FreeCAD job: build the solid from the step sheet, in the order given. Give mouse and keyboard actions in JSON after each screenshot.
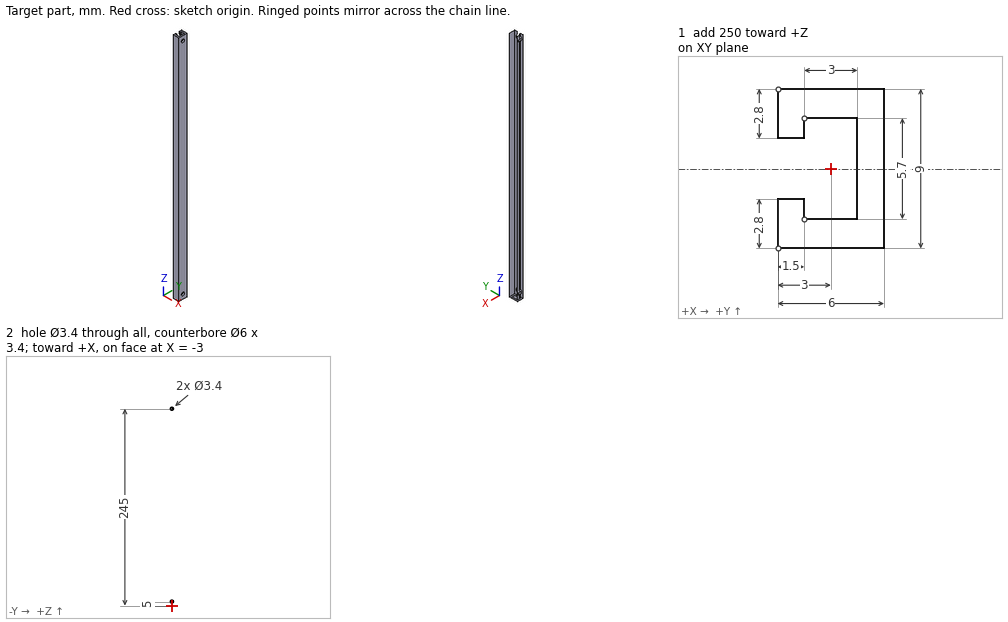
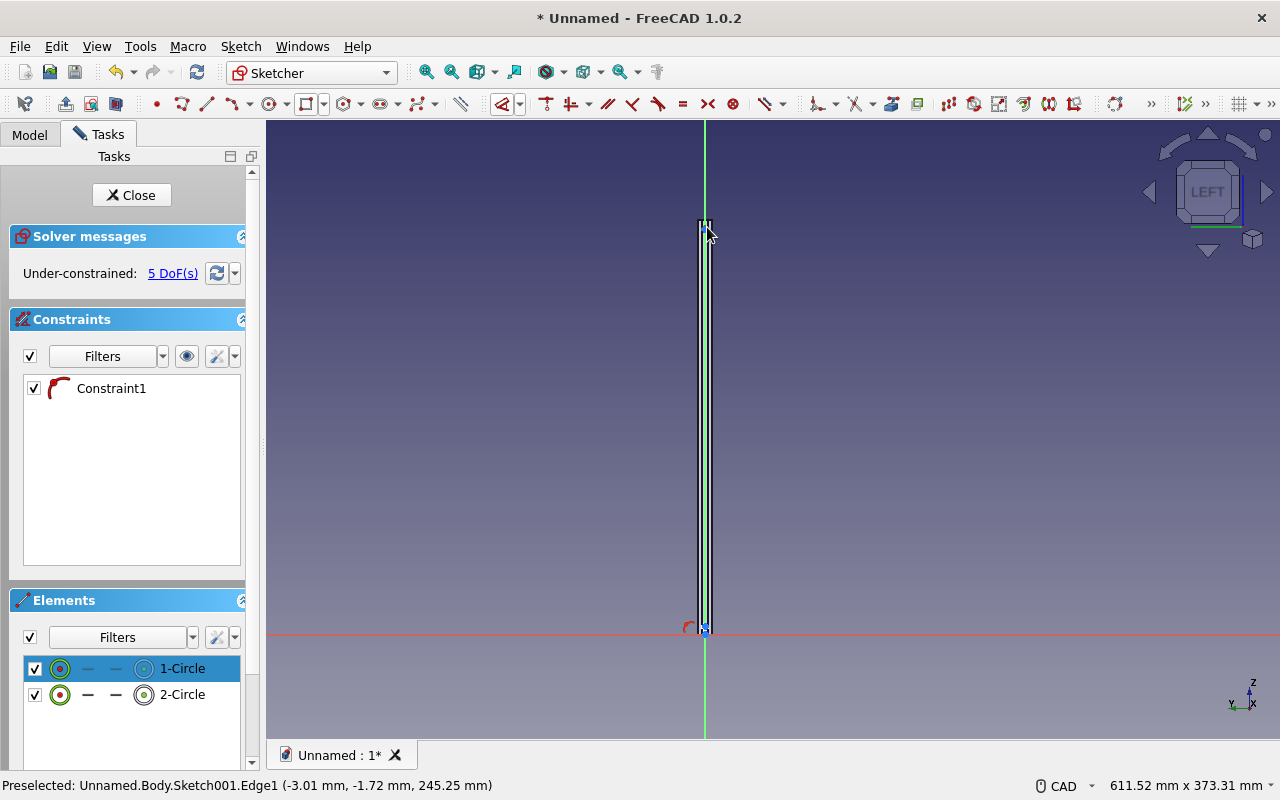
{"action": "scroll", "coordinate": [707, 625], "scroll_direction": "up", "scroll_amount": 10}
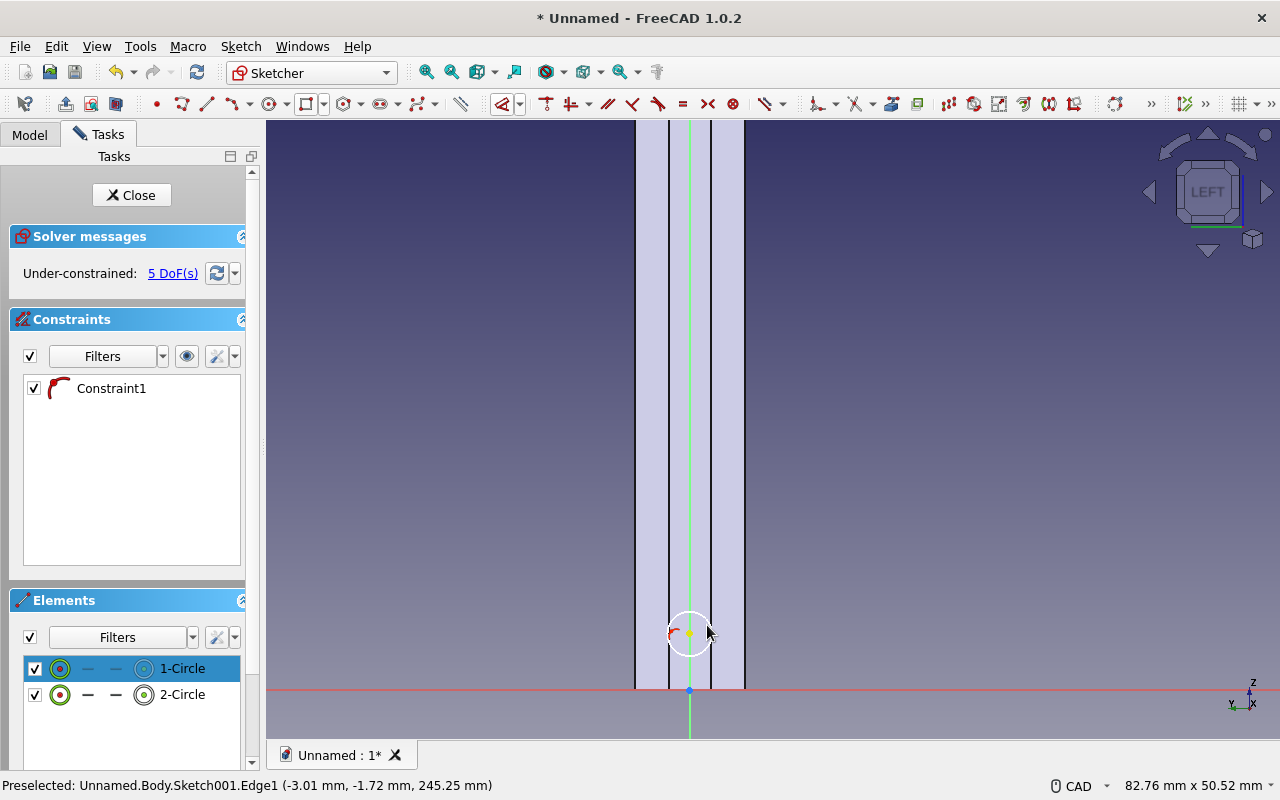
{"action": "left_click", "coordinate": [705, 618]}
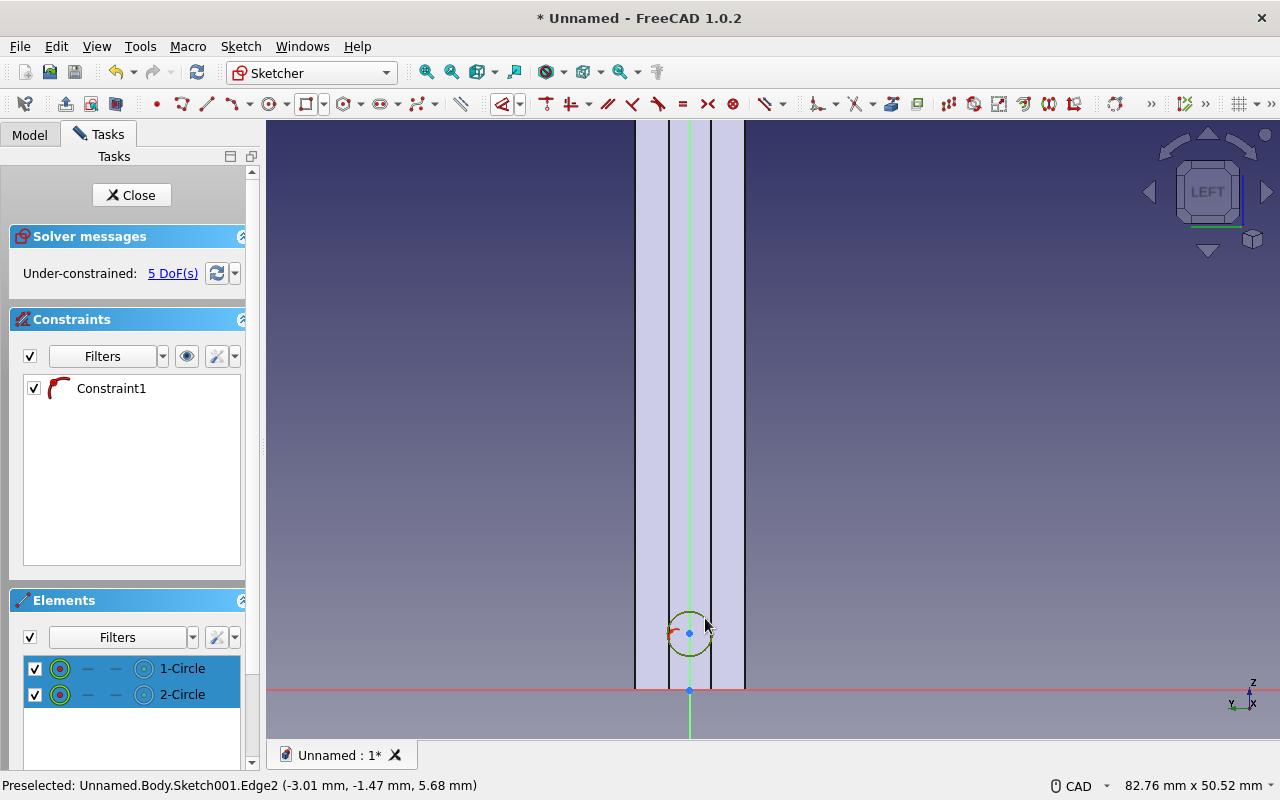
{"action": "left_click", "coordinate": [683, 104]}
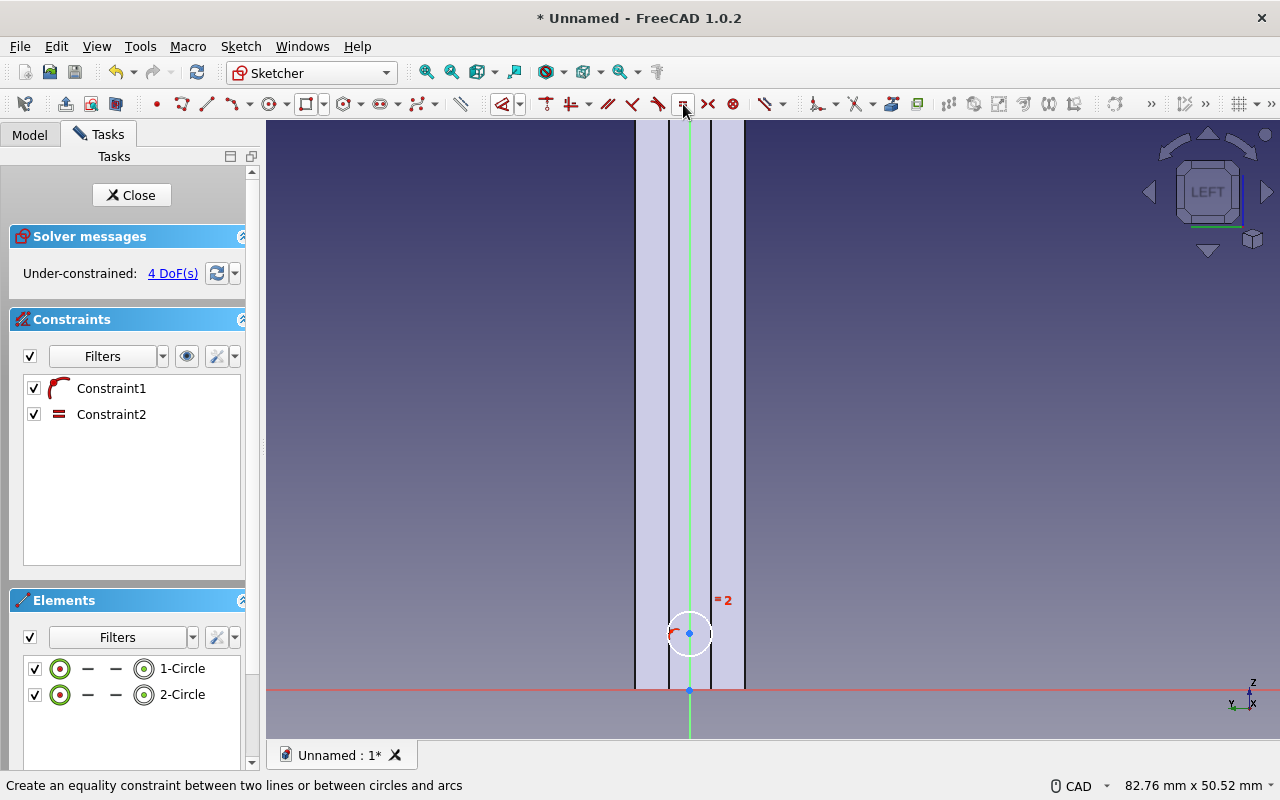
{"action": "scroll", "coordinate": [707, 625], "scroll_direction": "down", "scroll_amount": 10}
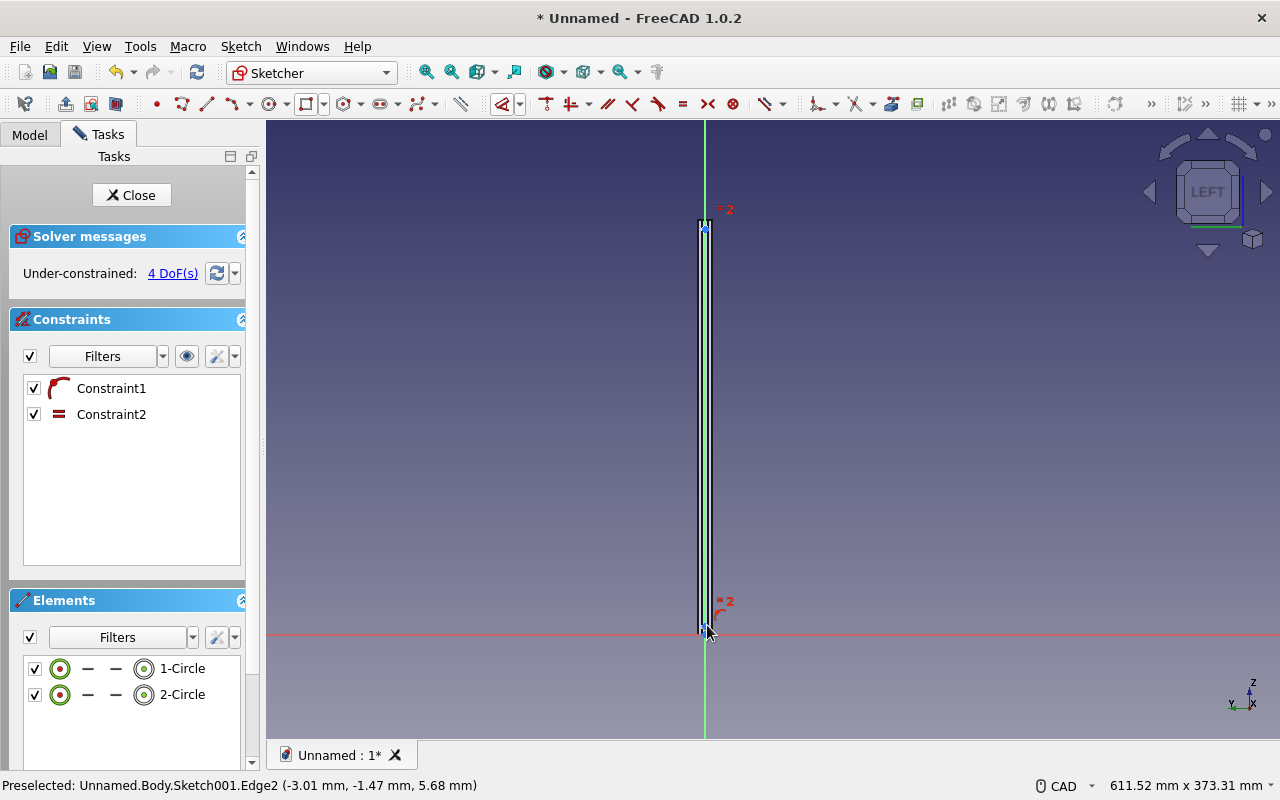
{"action": "left_click", "coordinate": [705, 229]}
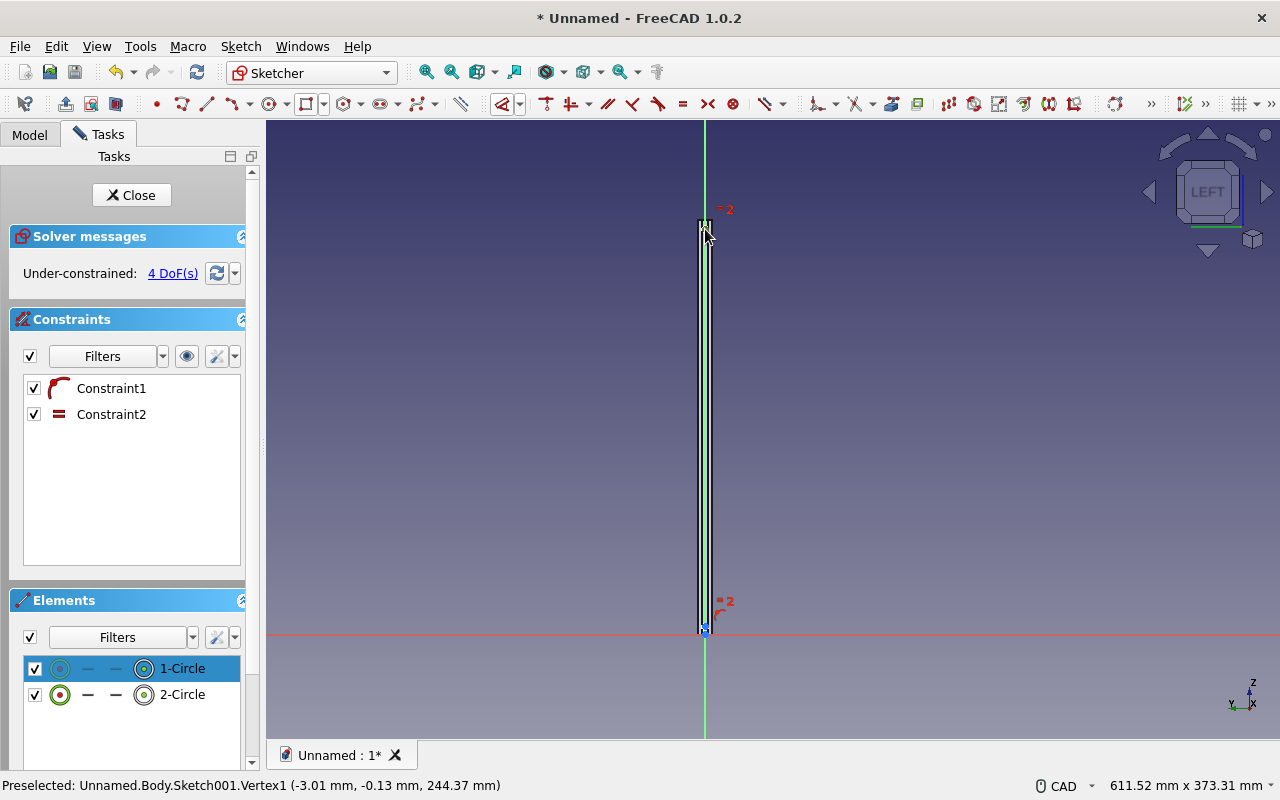
{"action": "left_click", "coordinate": [705, 671]}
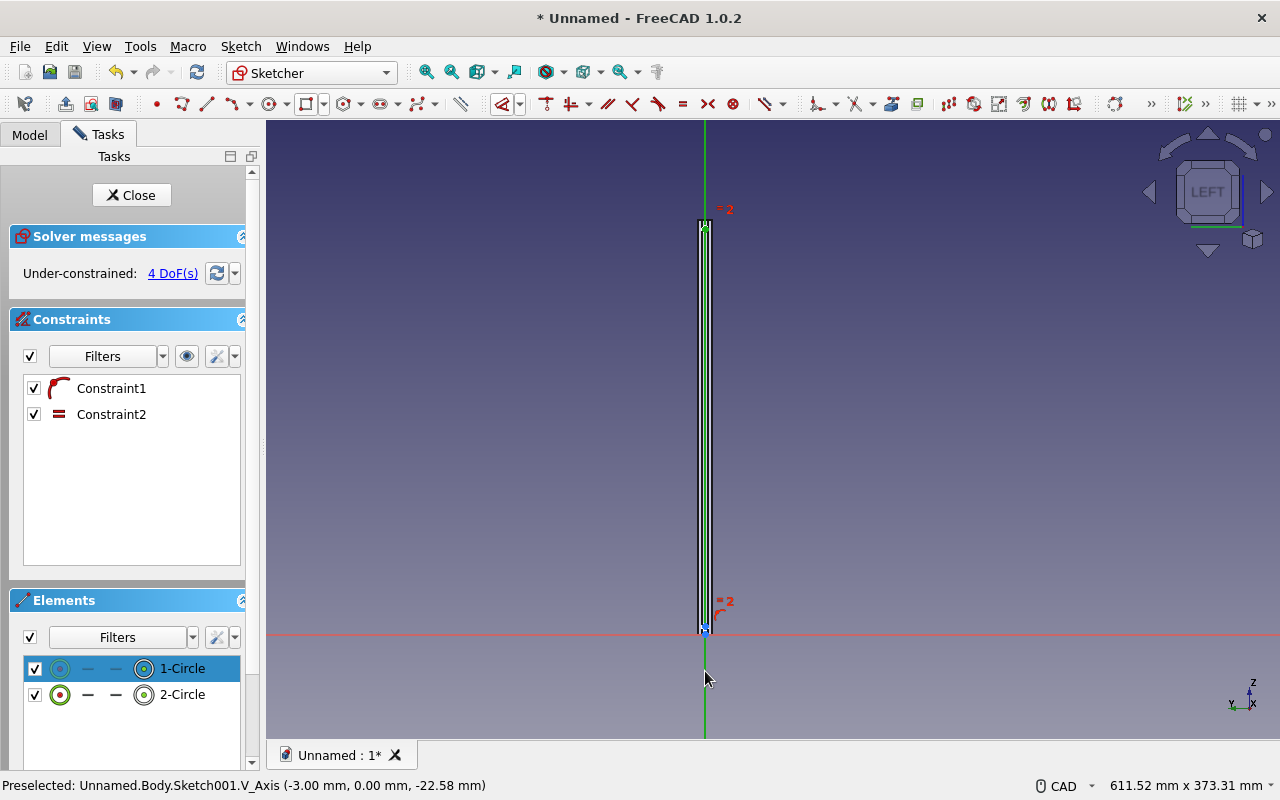
{"action": "left_click", "coordinate": [546, 104]}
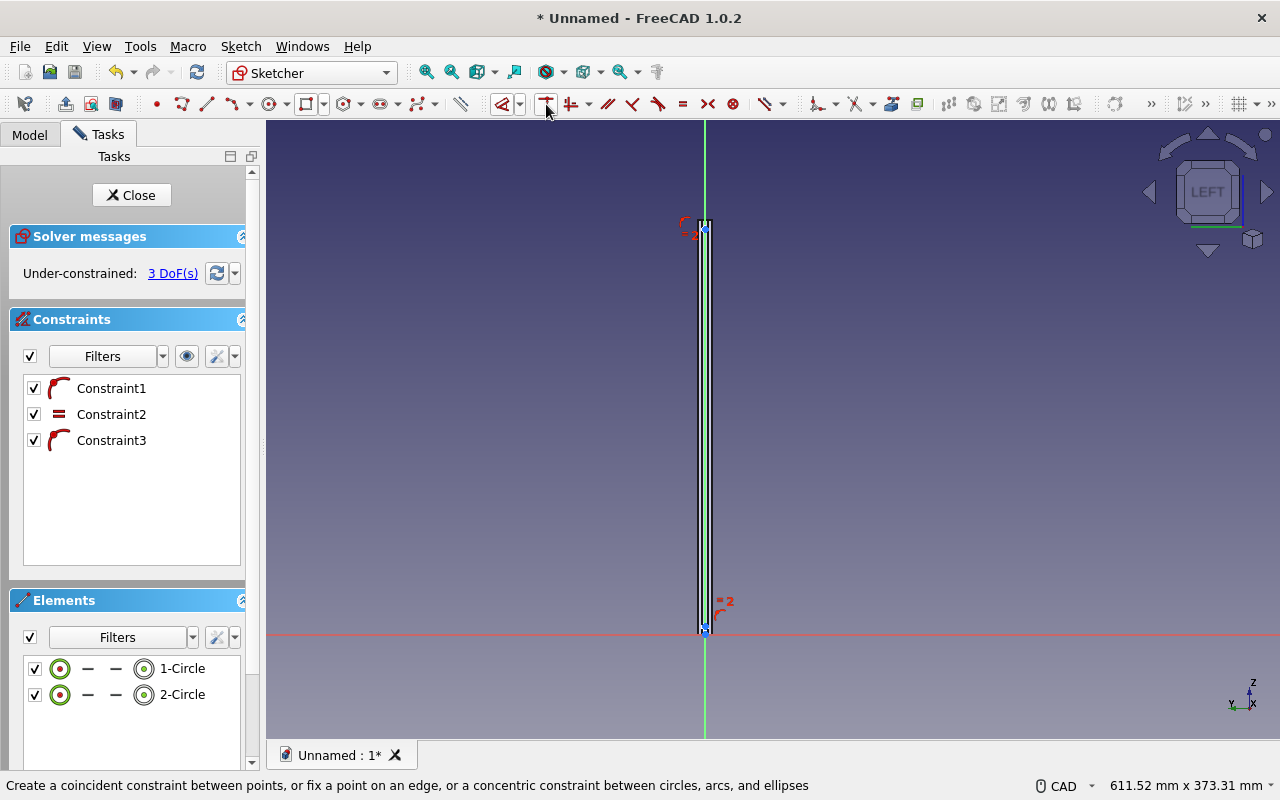
{"action": "left_click", "coordinate": [502, 104]}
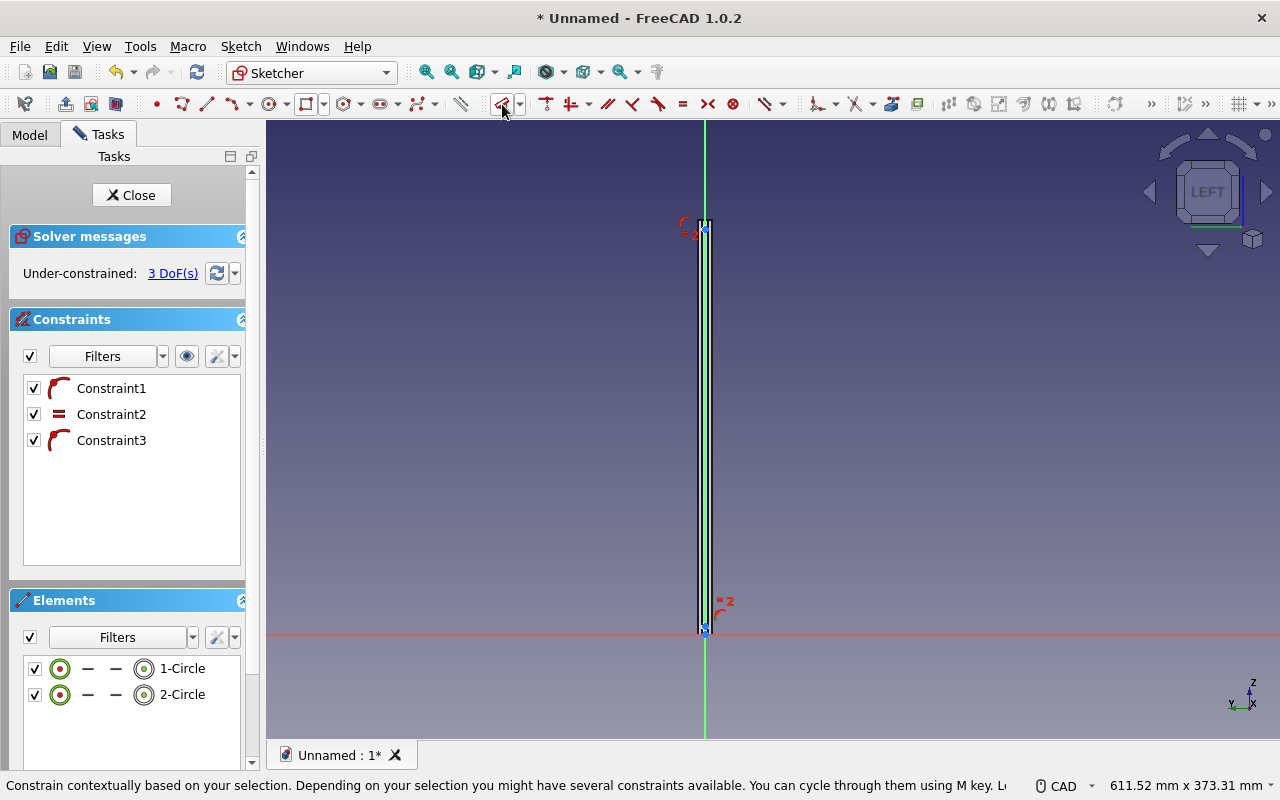
{"action": "scroll", "coordinate": [707, 227], "scroll_direction": "up", "scroll_amount": 10}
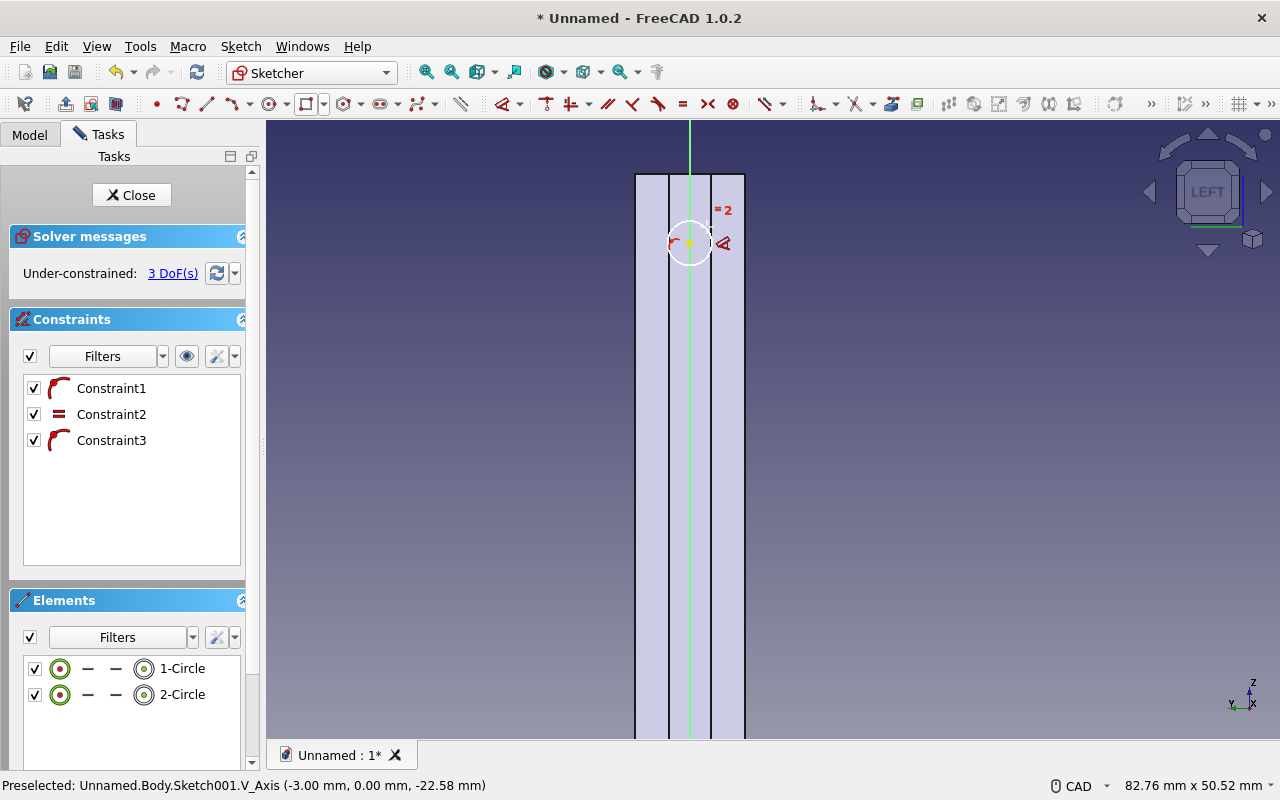
{"action": "left_click", "coordinate": [705, 228]}
{"action": "left_click", "coordinate": [728, 205]}